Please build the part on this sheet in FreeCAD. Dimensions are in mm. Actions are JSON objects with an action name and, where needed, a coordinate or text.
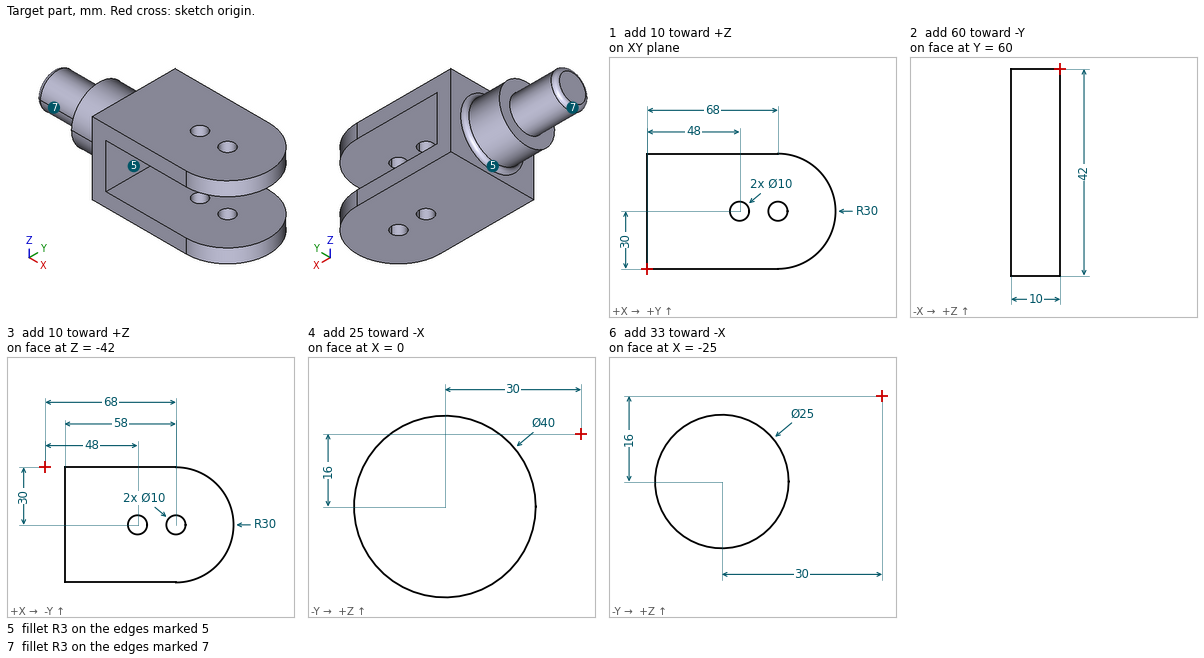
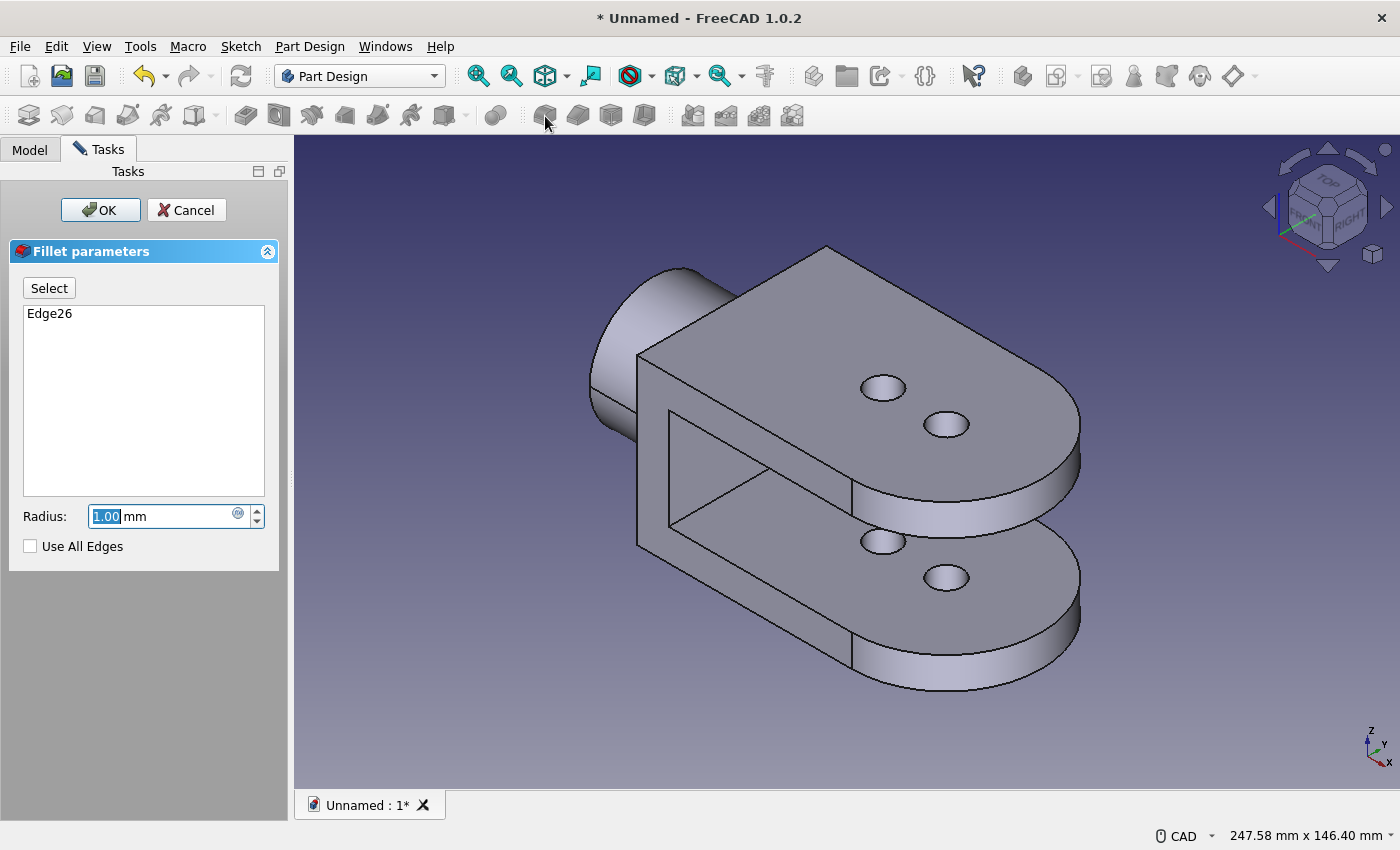
{"action": "type", "text": "3"}
{"action": "key", "text": "Tab"}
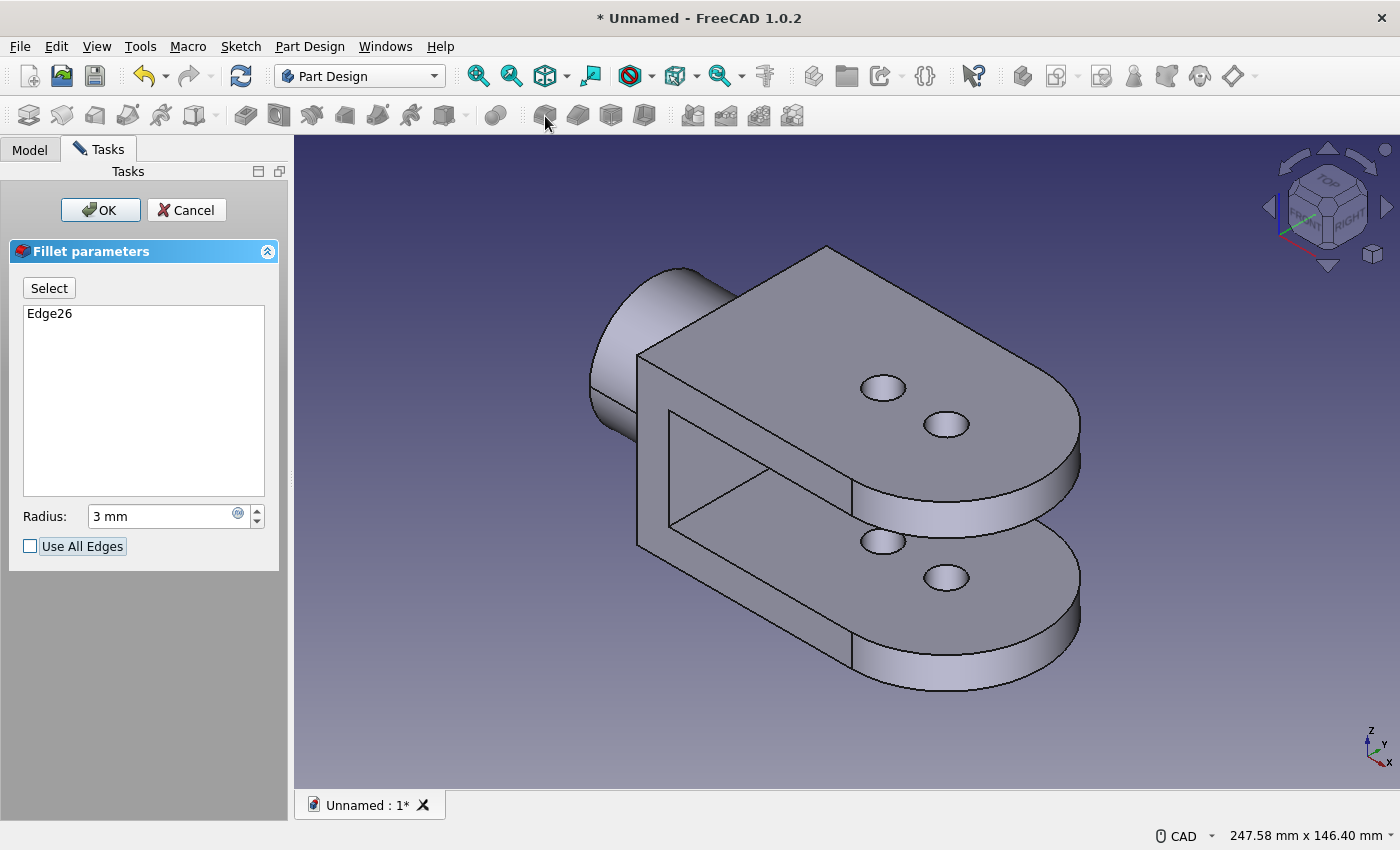
{"action": "left_click", "coordinate": [101, 210]}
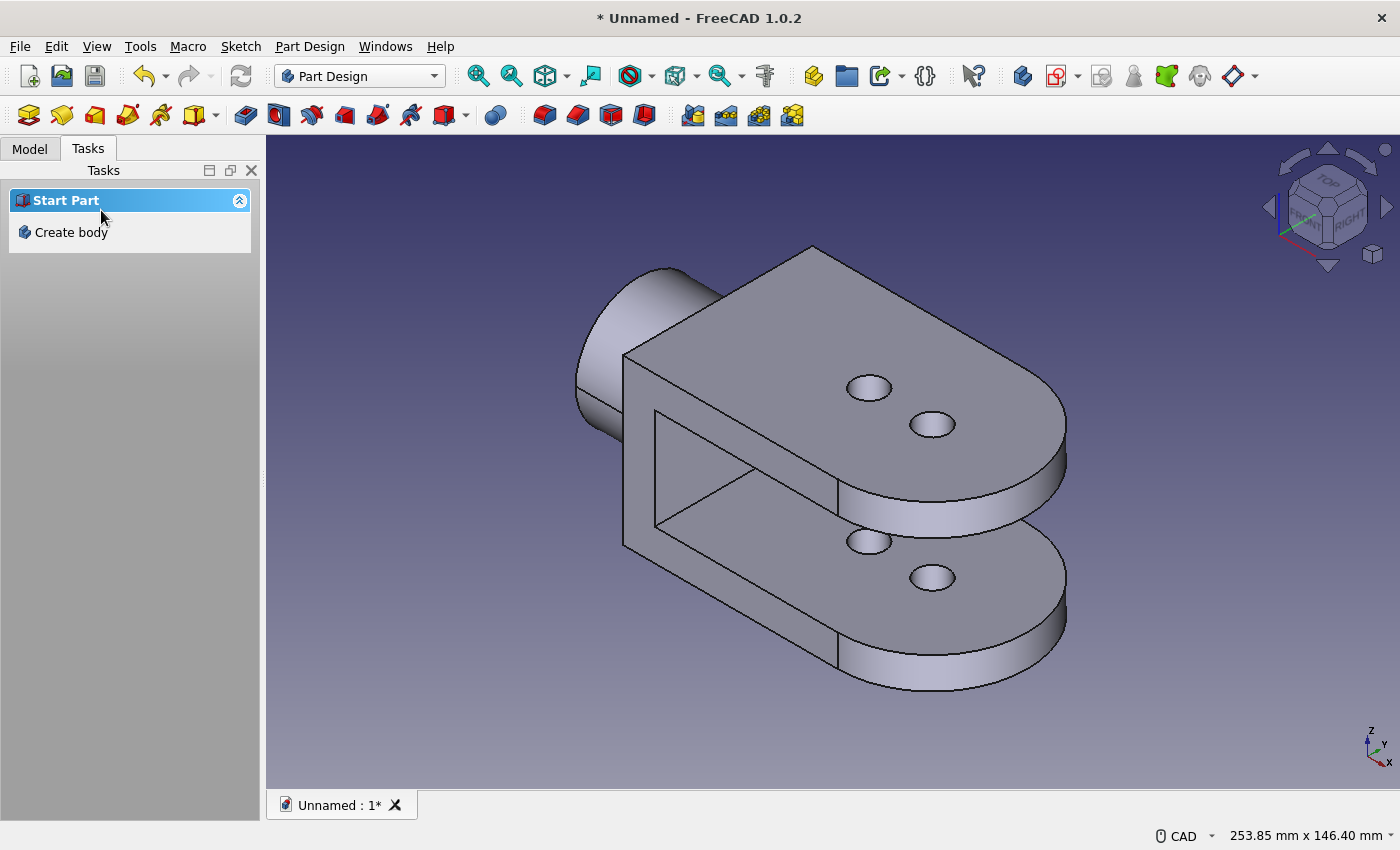
{"action": "key", "text": "6"}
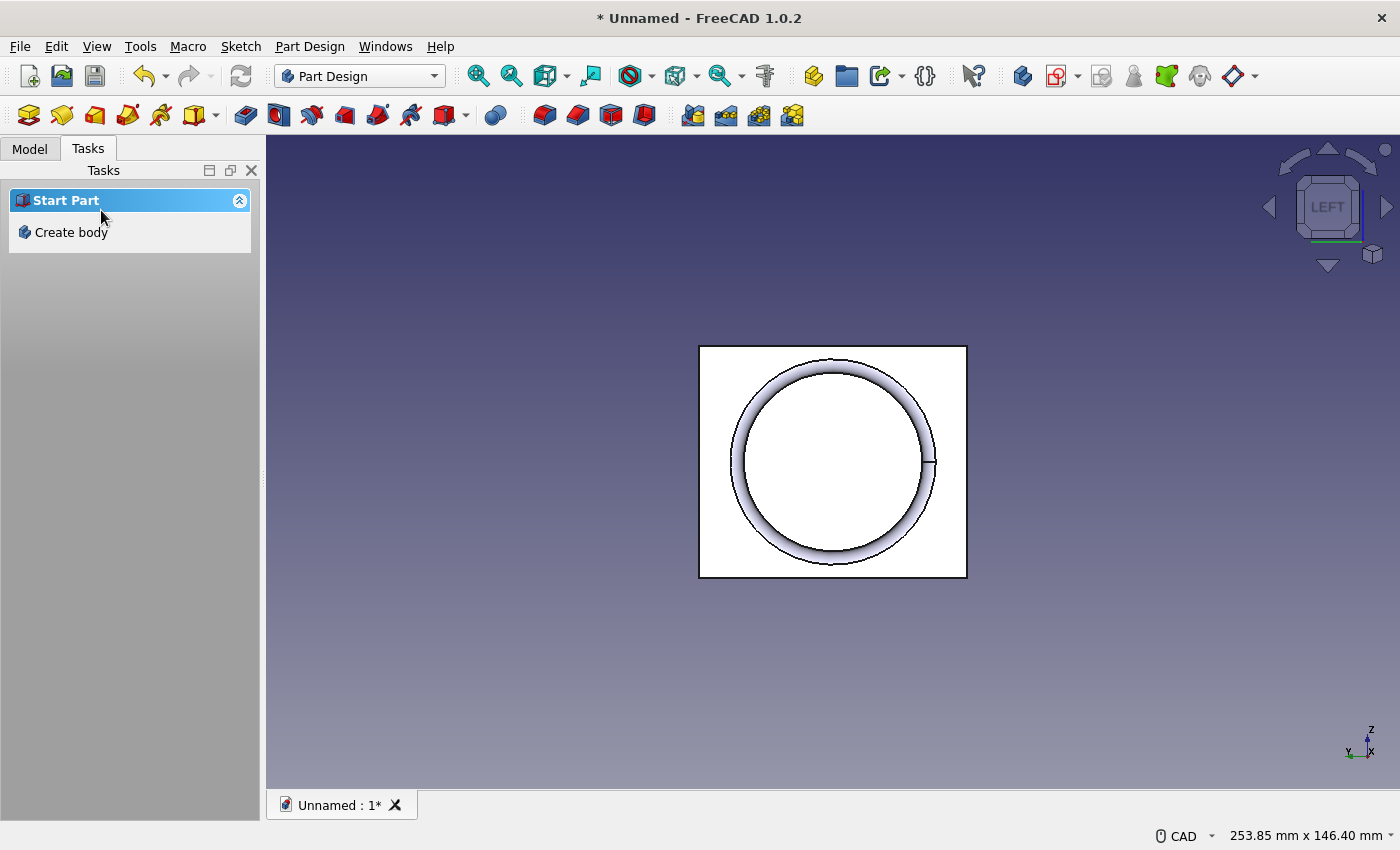
{"action": "key", "text": "v f"}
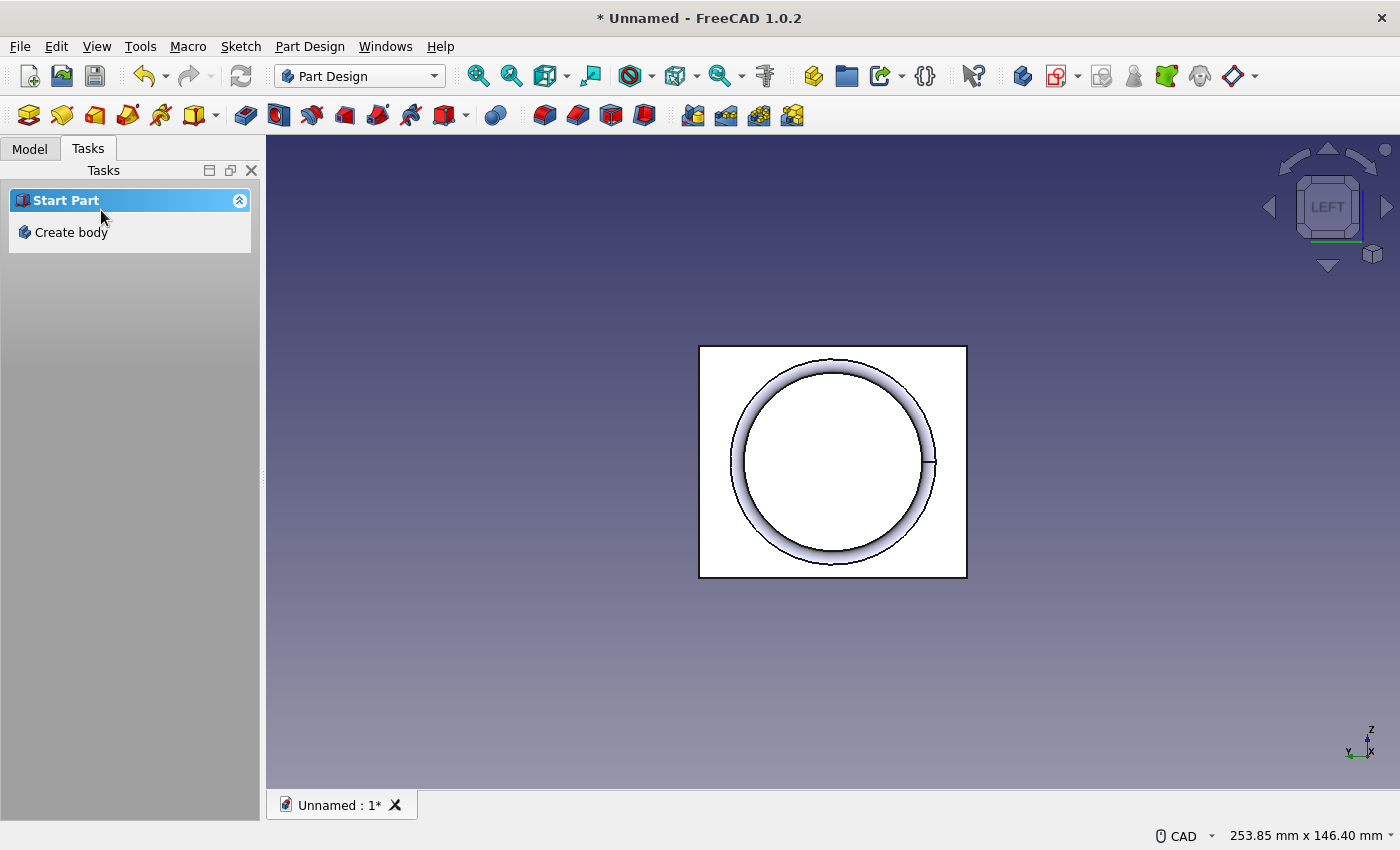
{"action": "left_click", "coordinate": [833, 461]}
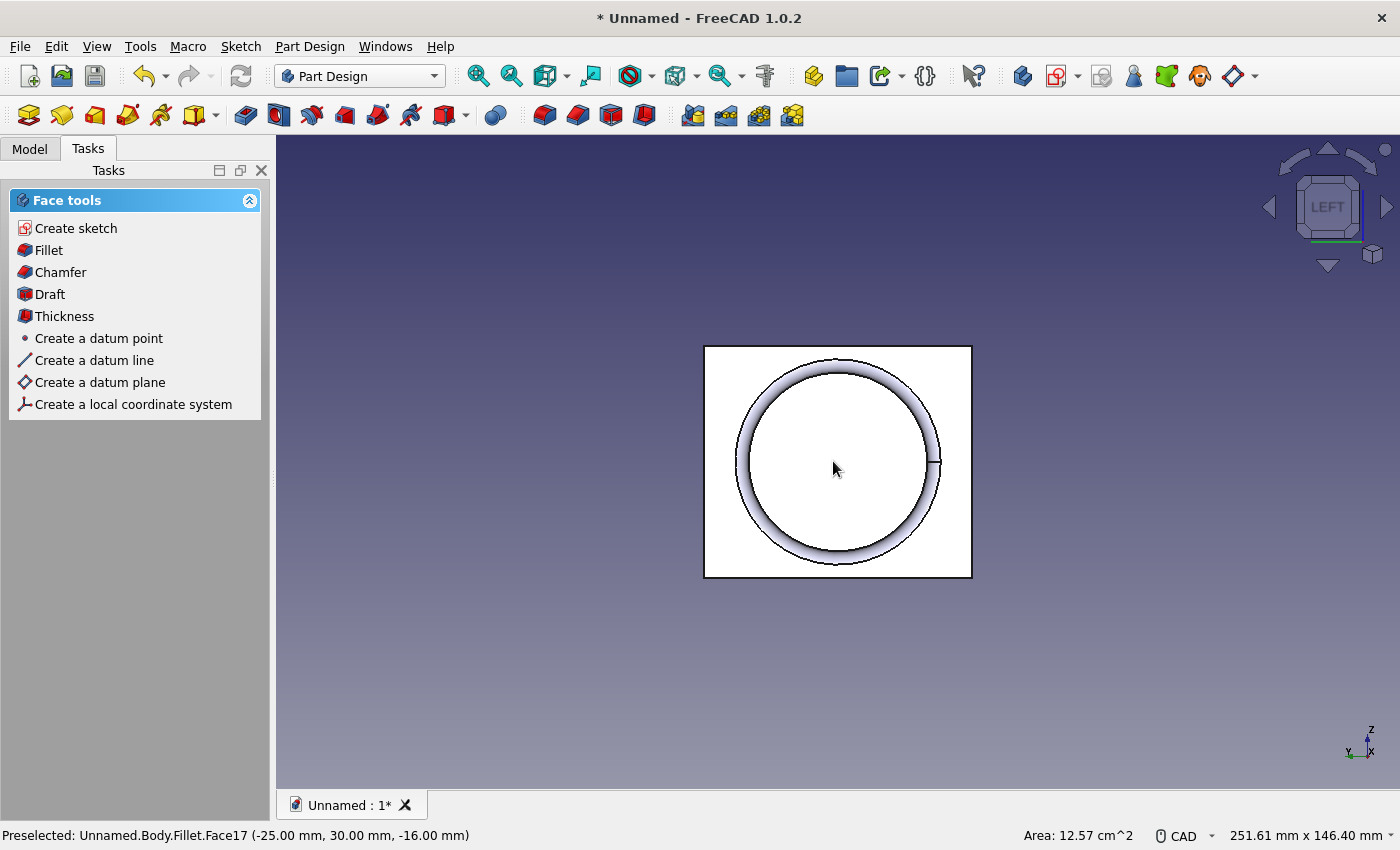
{"action": "left_click", "coordinate": [1056, 76]}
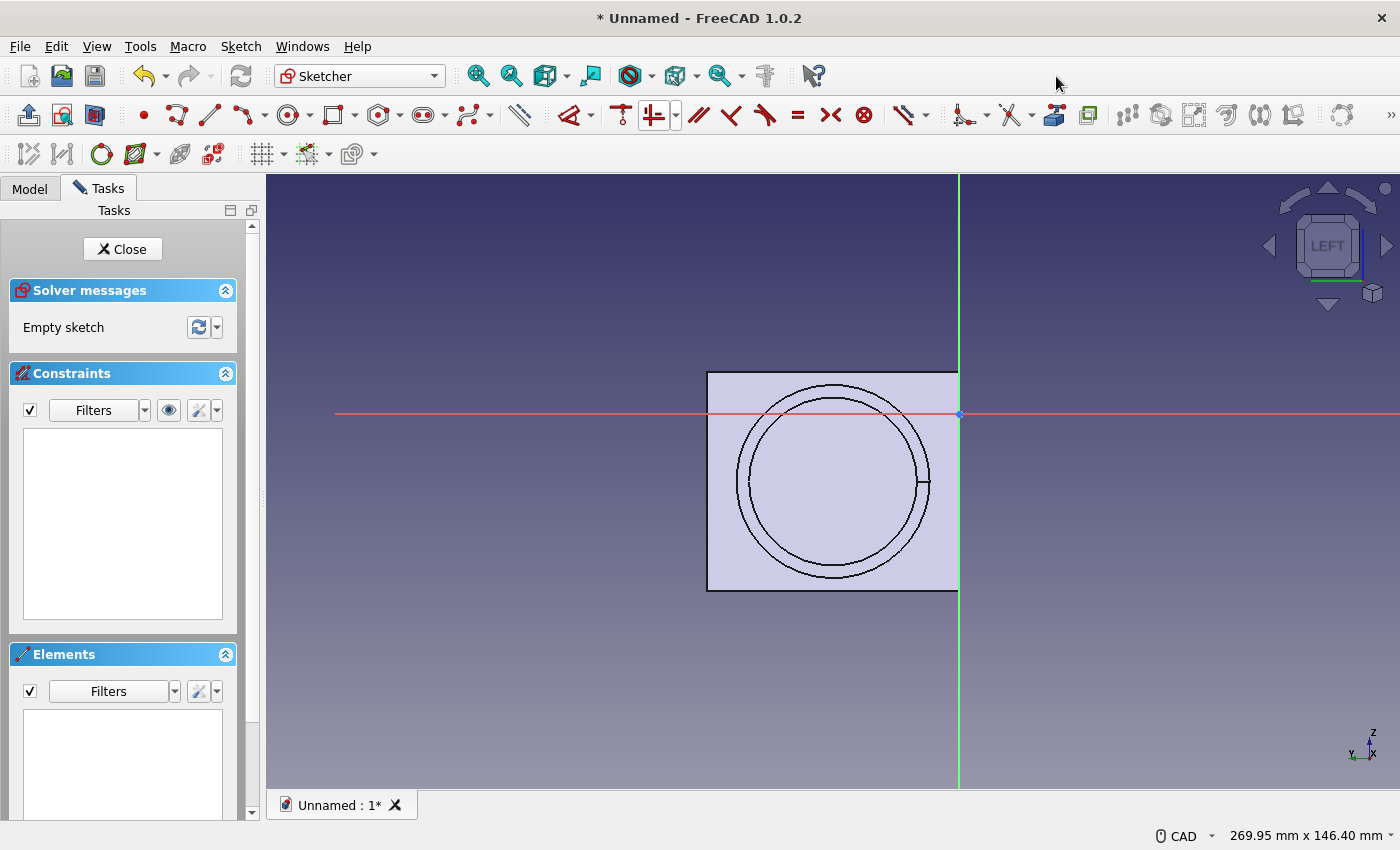
{"action": "scroll", "coordinate": [915, 471], "scroll_direction": "up", "scroll_amount": 6}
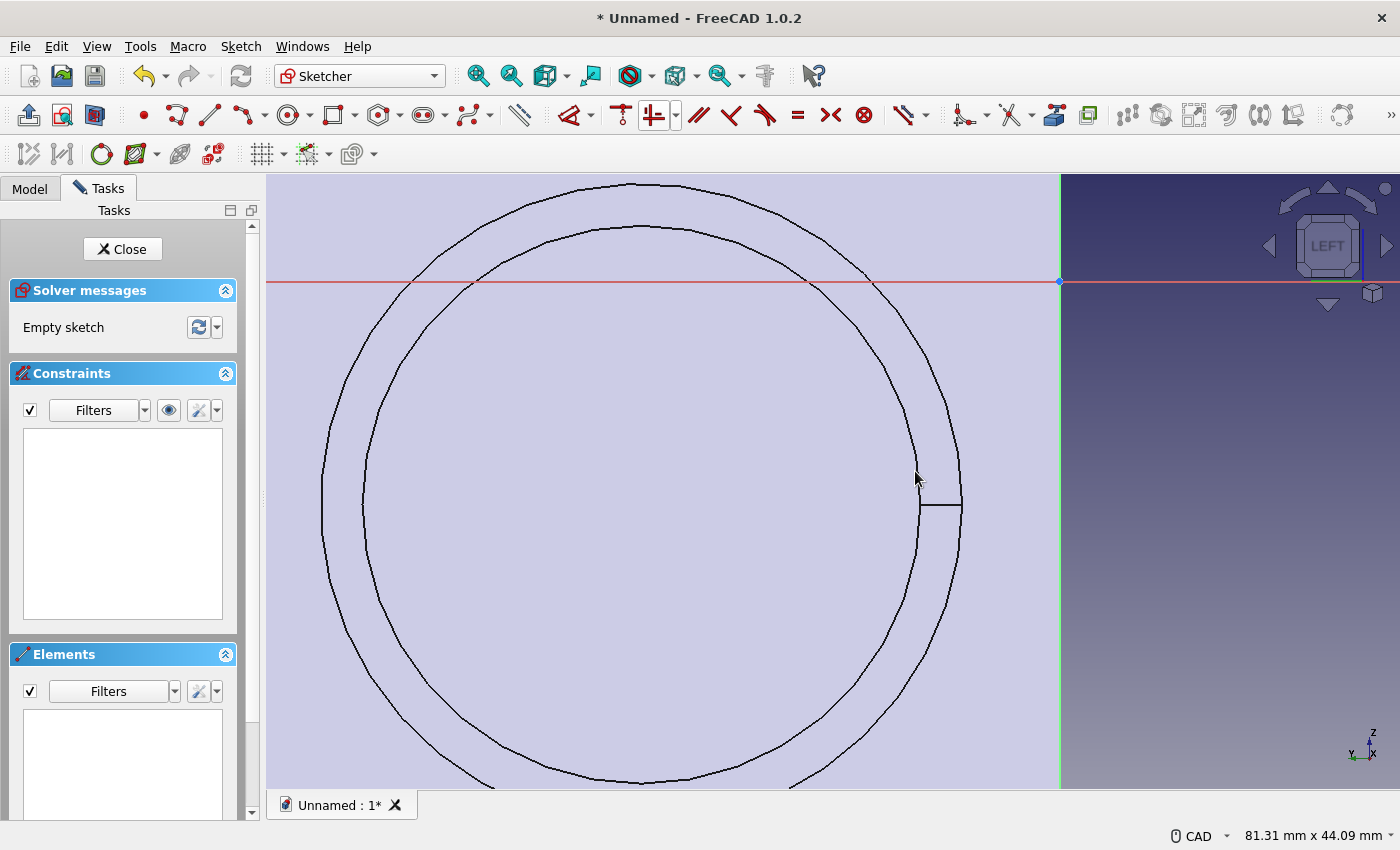
{"action": "left_click", "coordinate": [288, 116]}